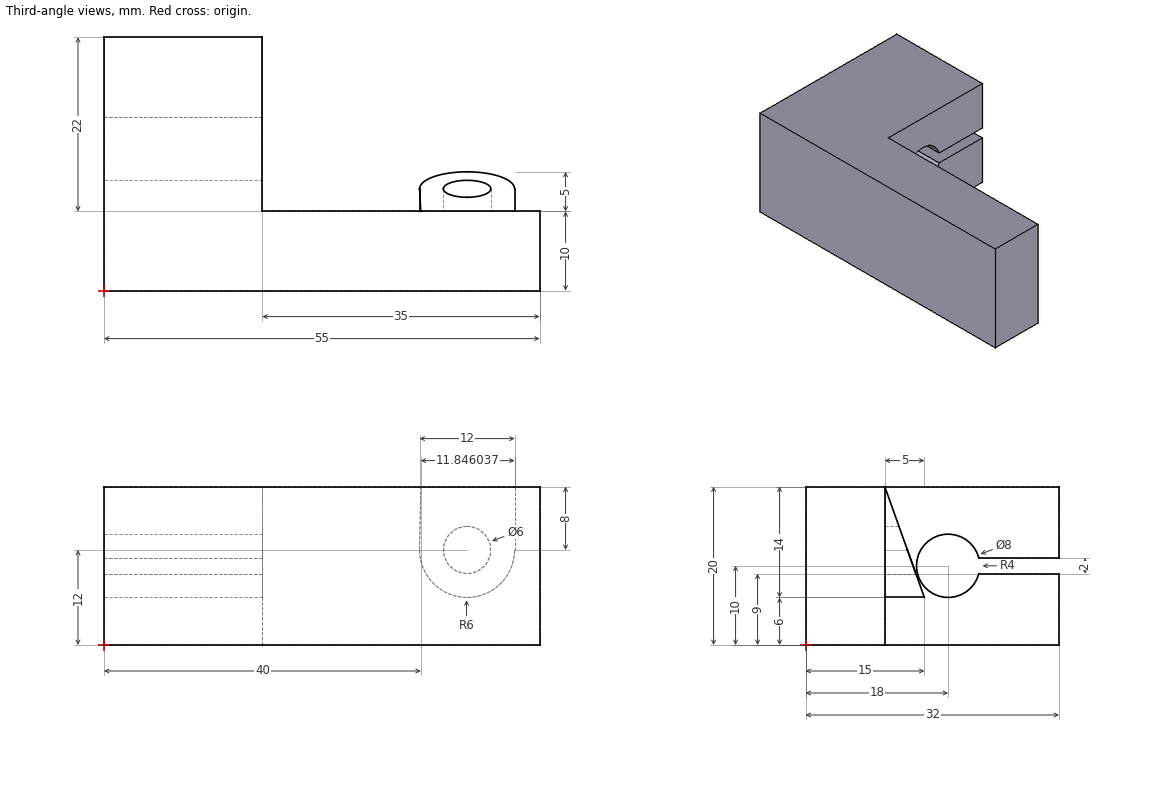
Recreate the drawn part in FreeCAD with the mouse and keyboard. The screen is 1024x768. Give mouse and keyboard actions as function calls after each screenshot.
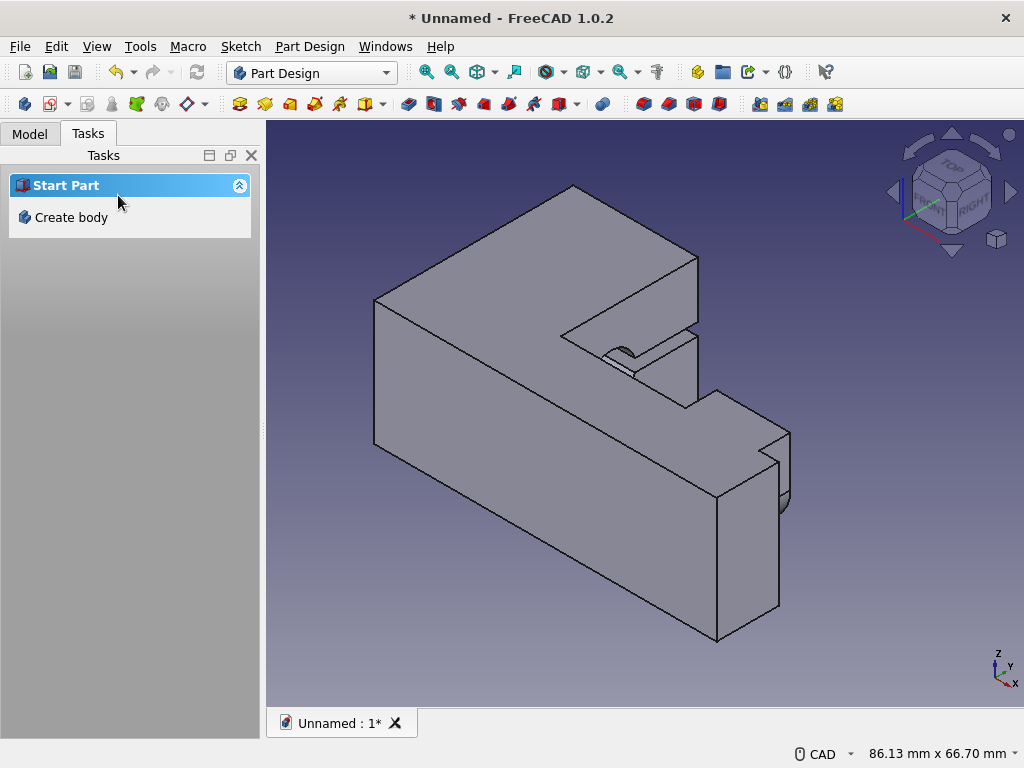
key(3)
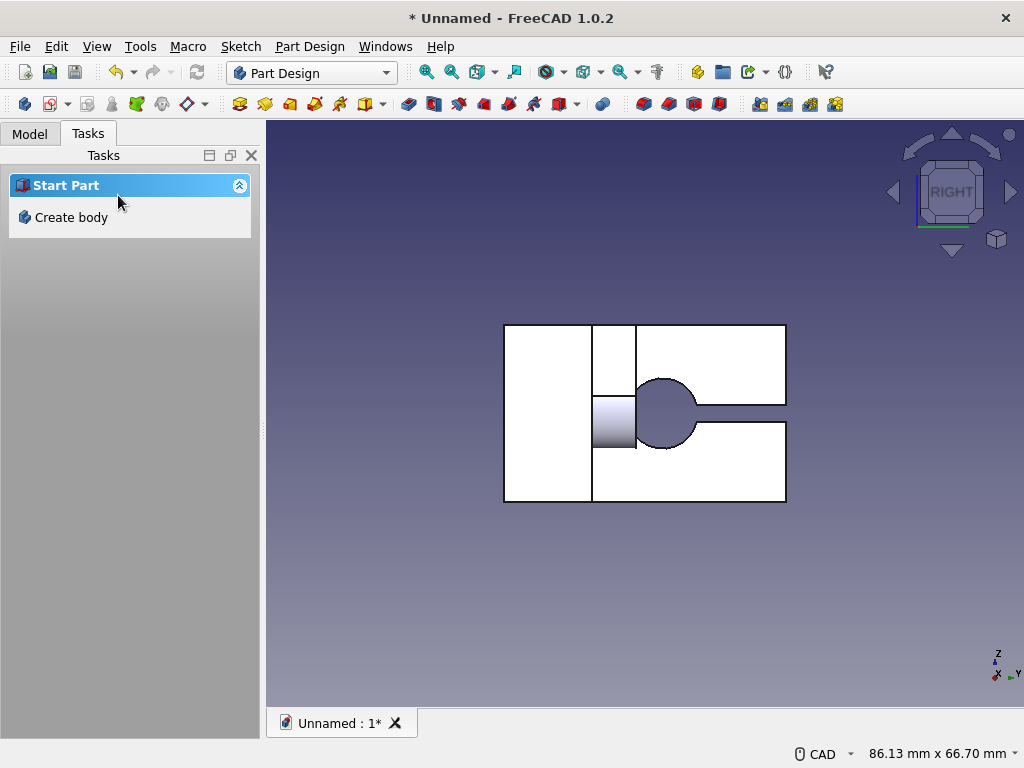
key(v)
key(f)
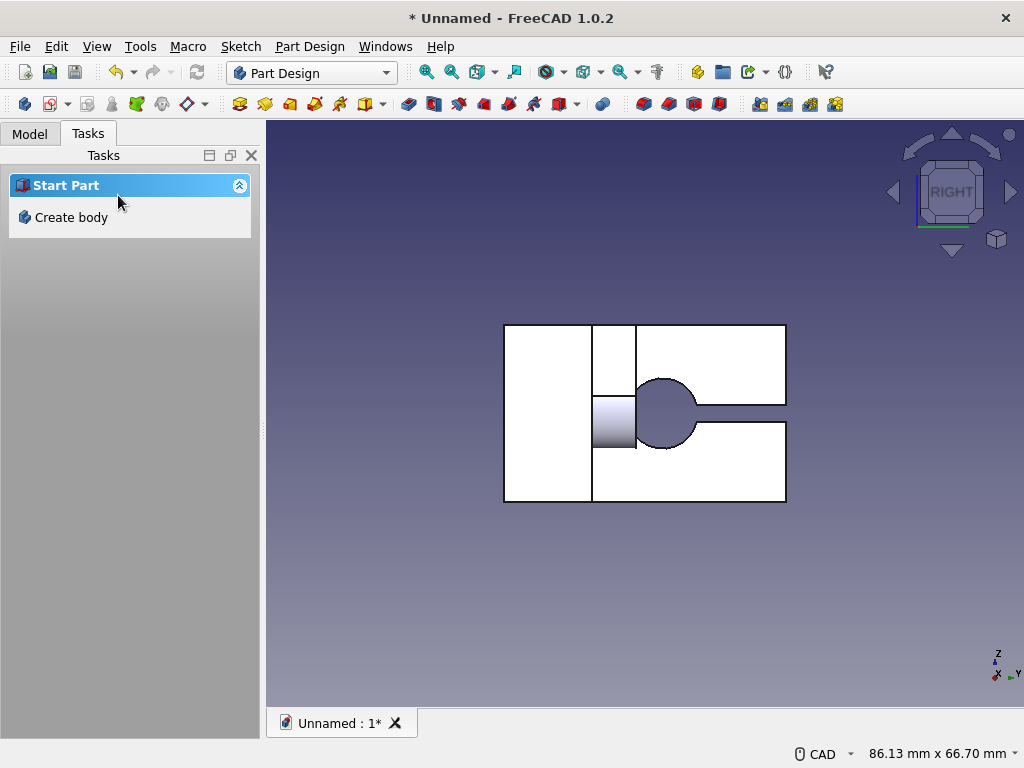
click(614, 350)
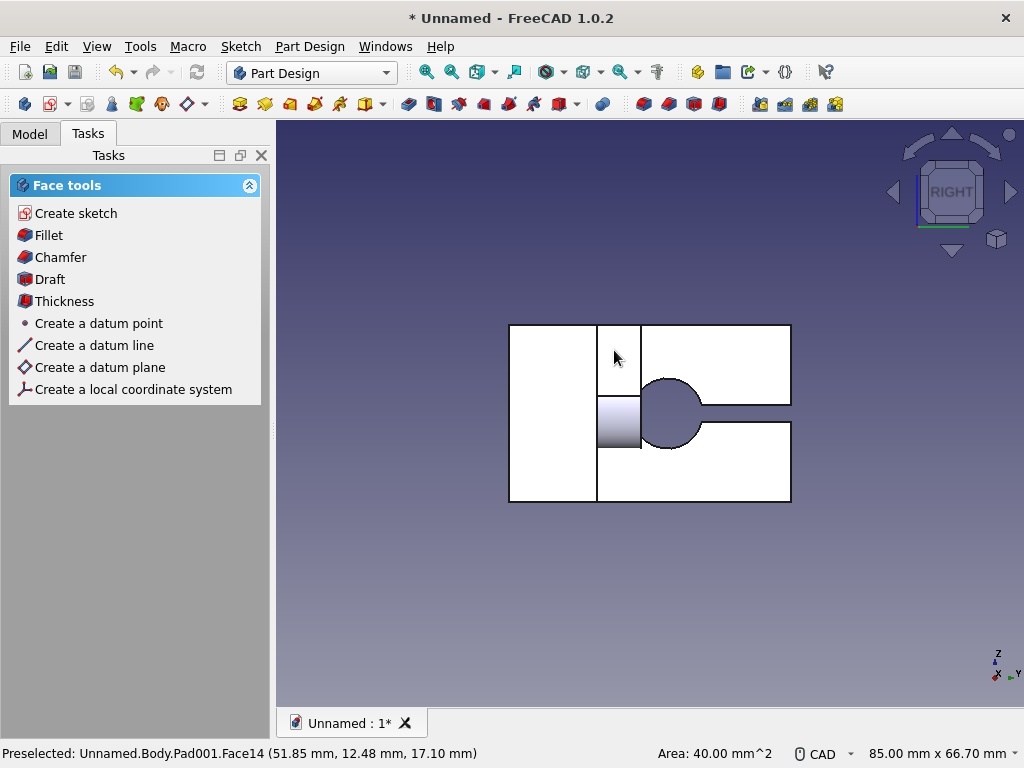
click(50, 104)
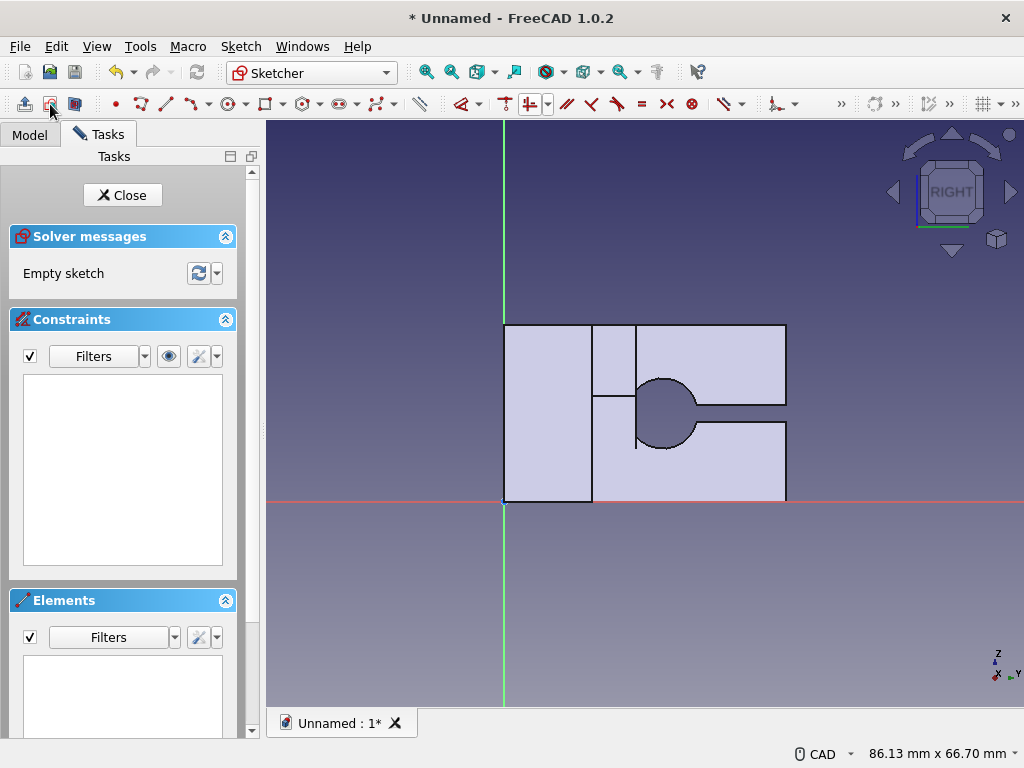
key(q)
key(s)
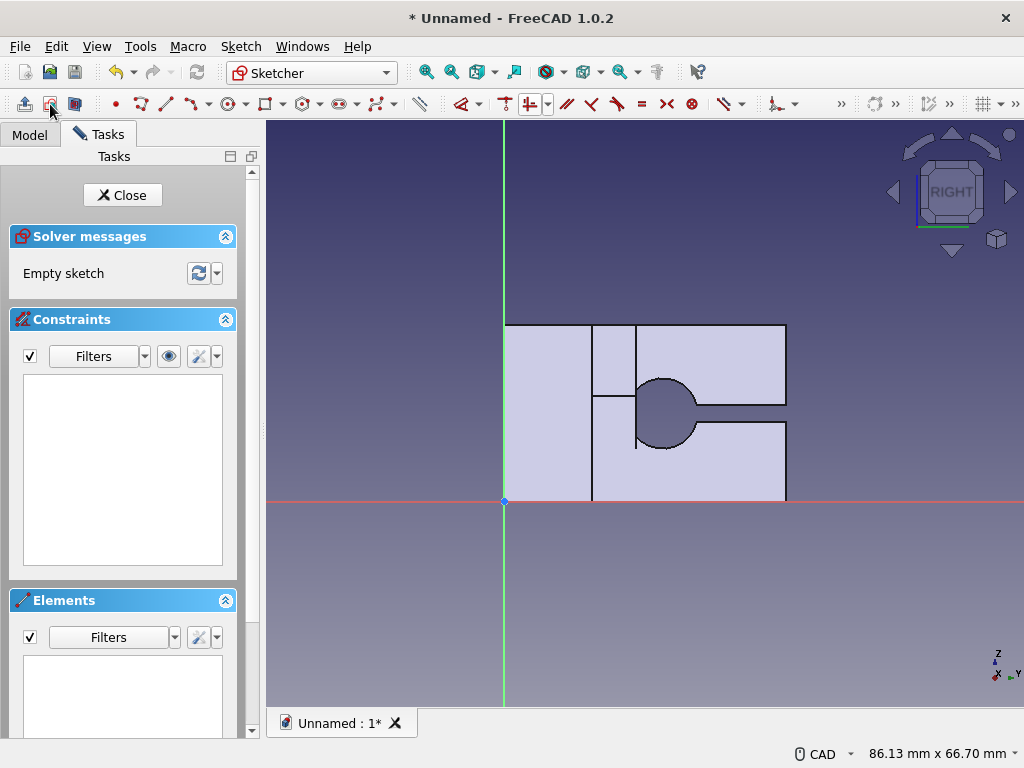
scroll(565, 413, up, 4)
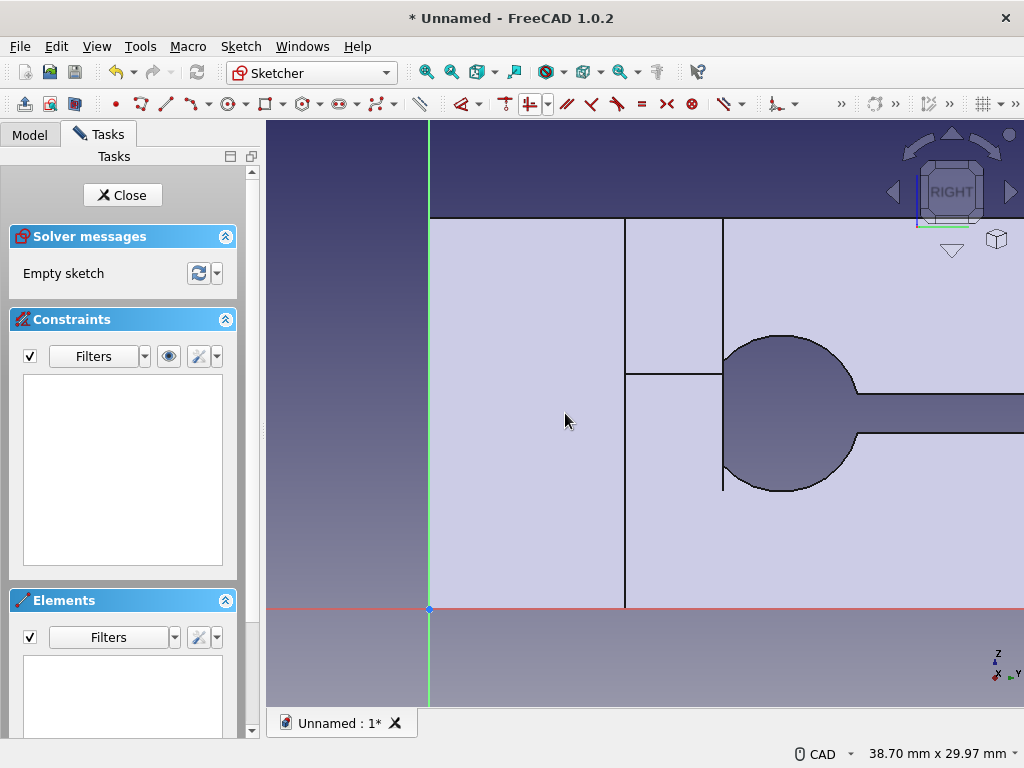
key(g)
key(m)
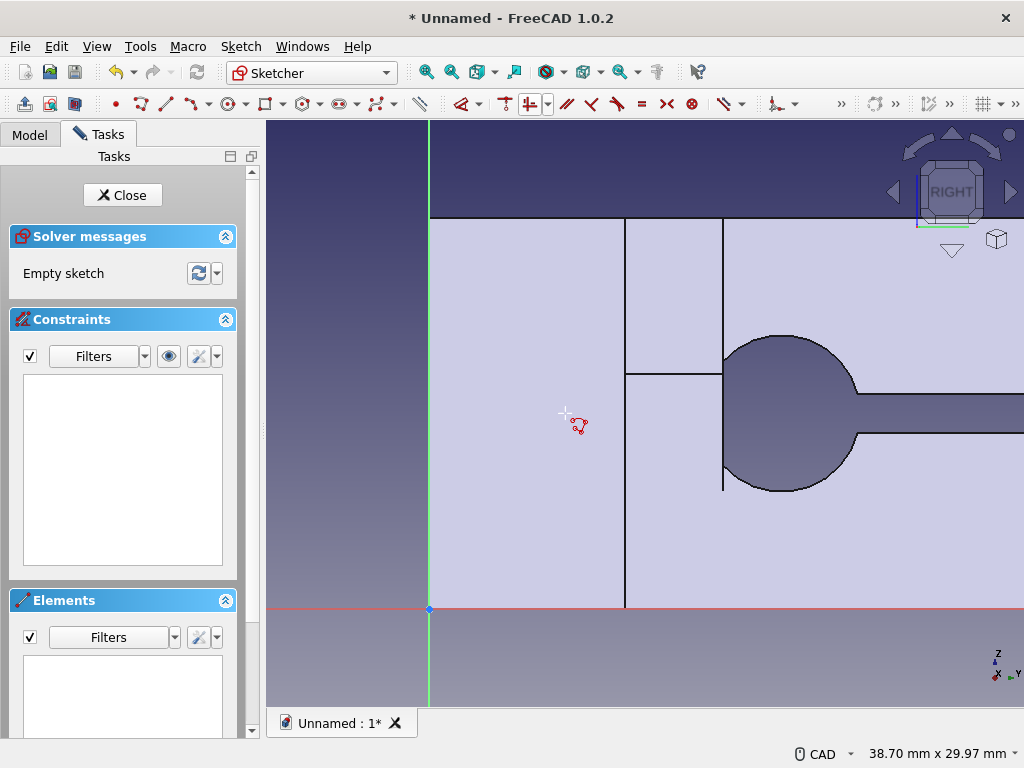
click(723, 492)
click(723, 218)
click(625, 218)
click(723, 493)
key(Escape)
key(Escape)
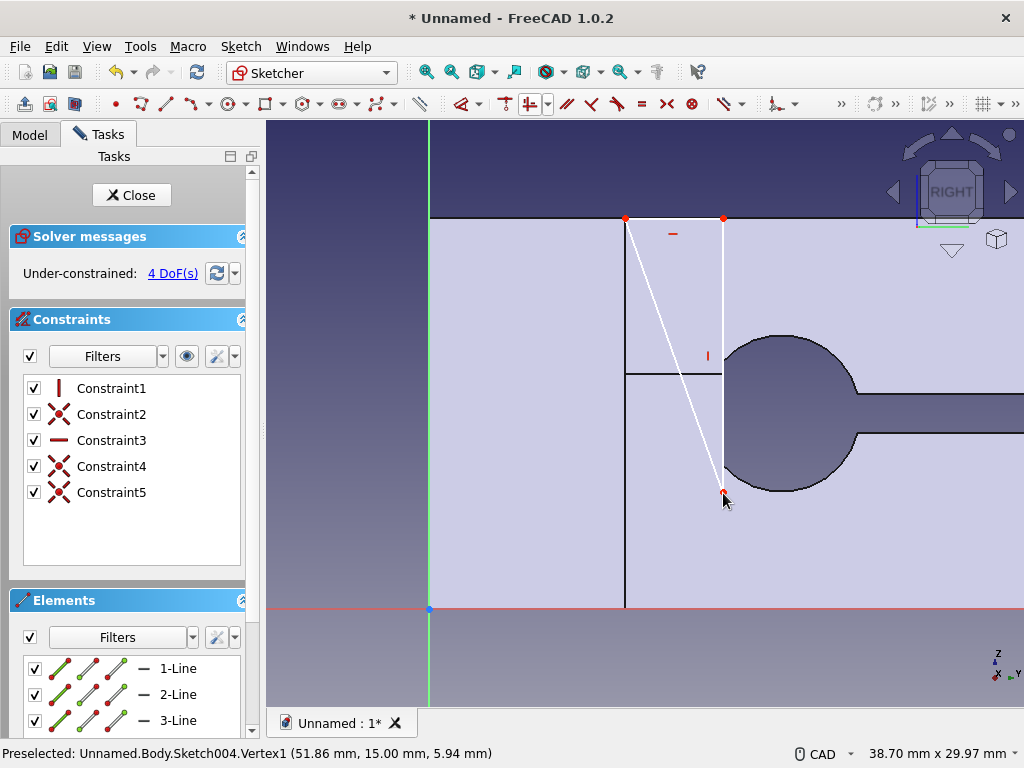
key(d)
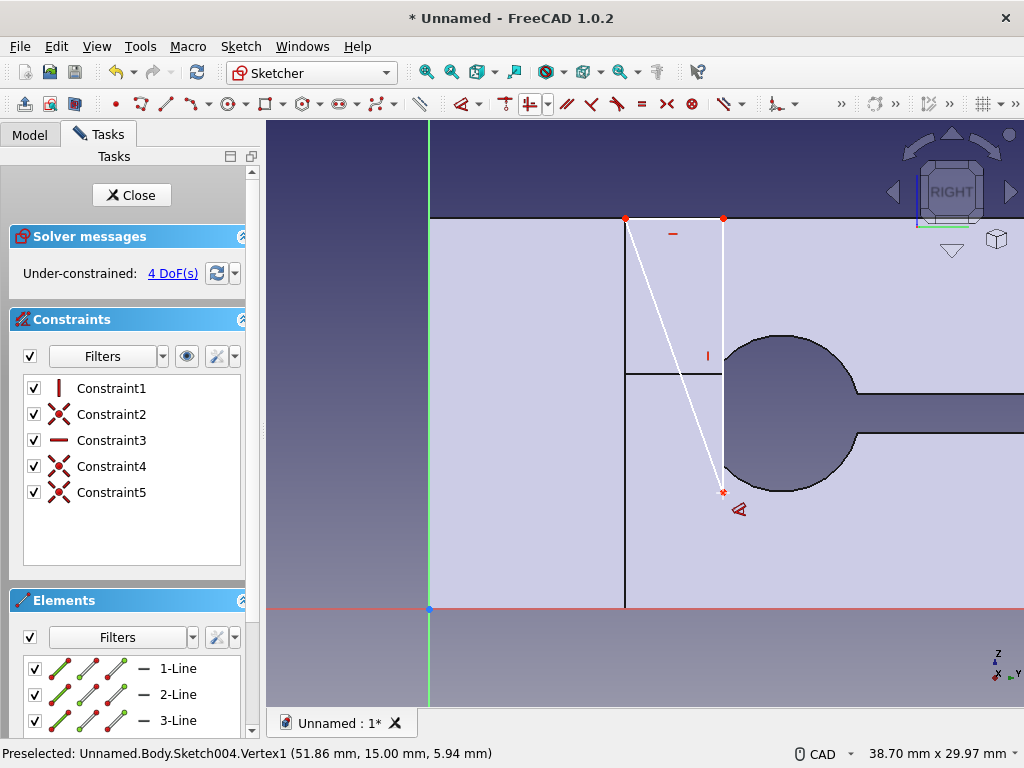
click(694, 219)
click(674, 185)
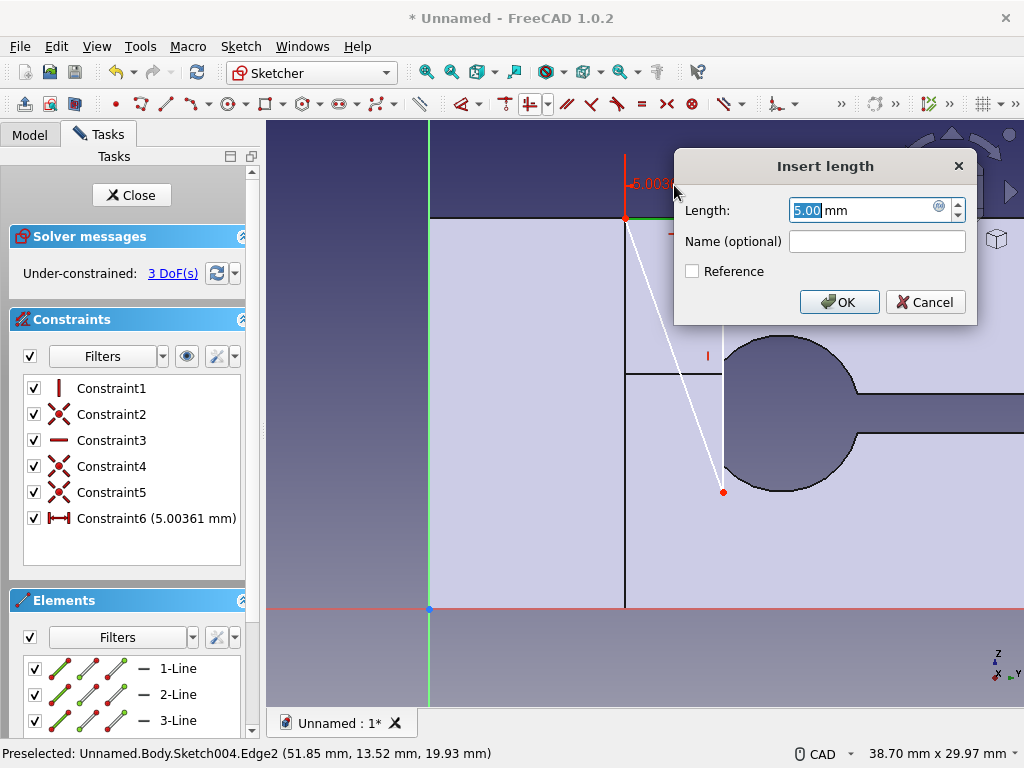
text(5)
key(Return)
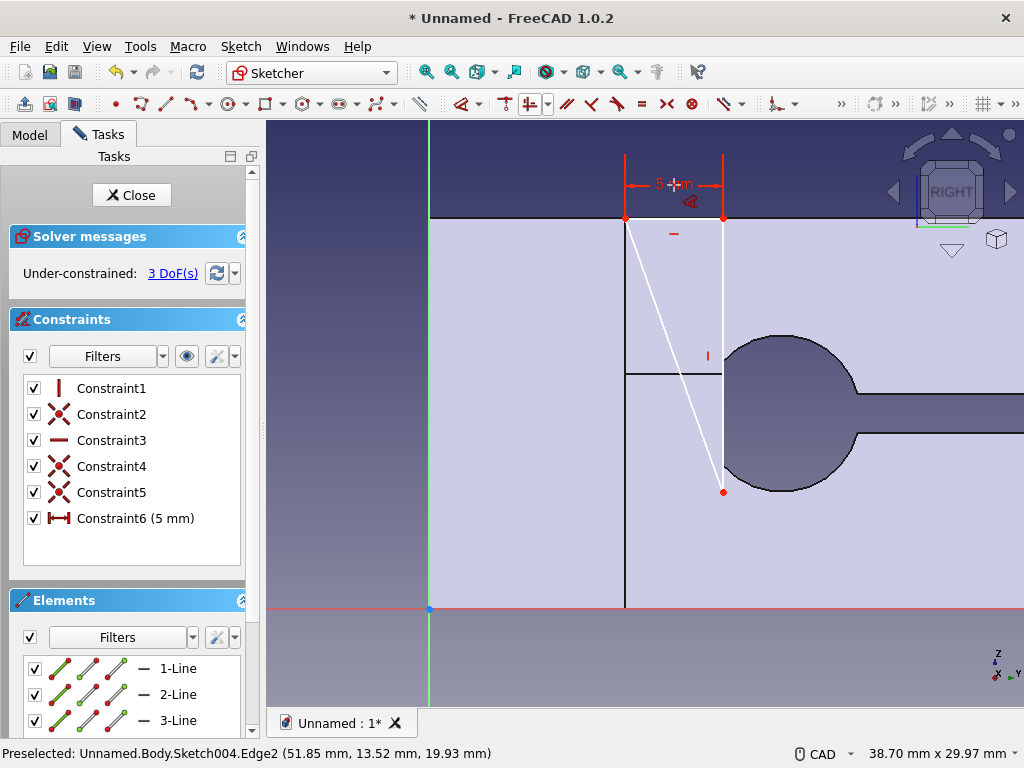
click(723, 411)
click(757, 356)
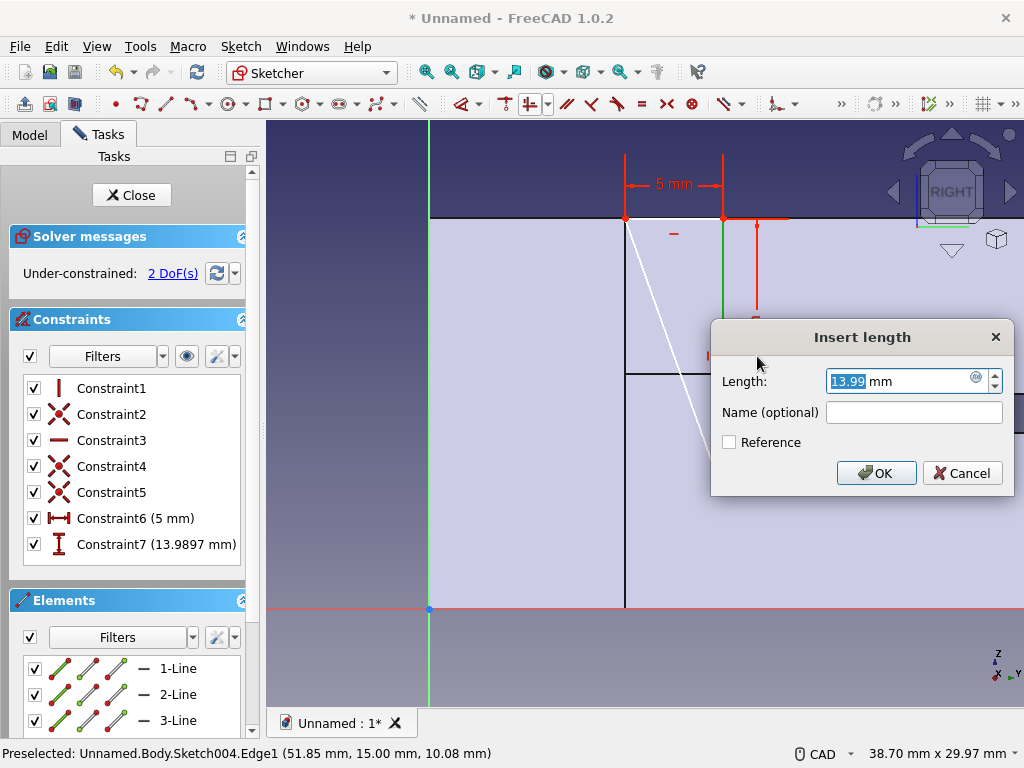
text(14)
key(Return)